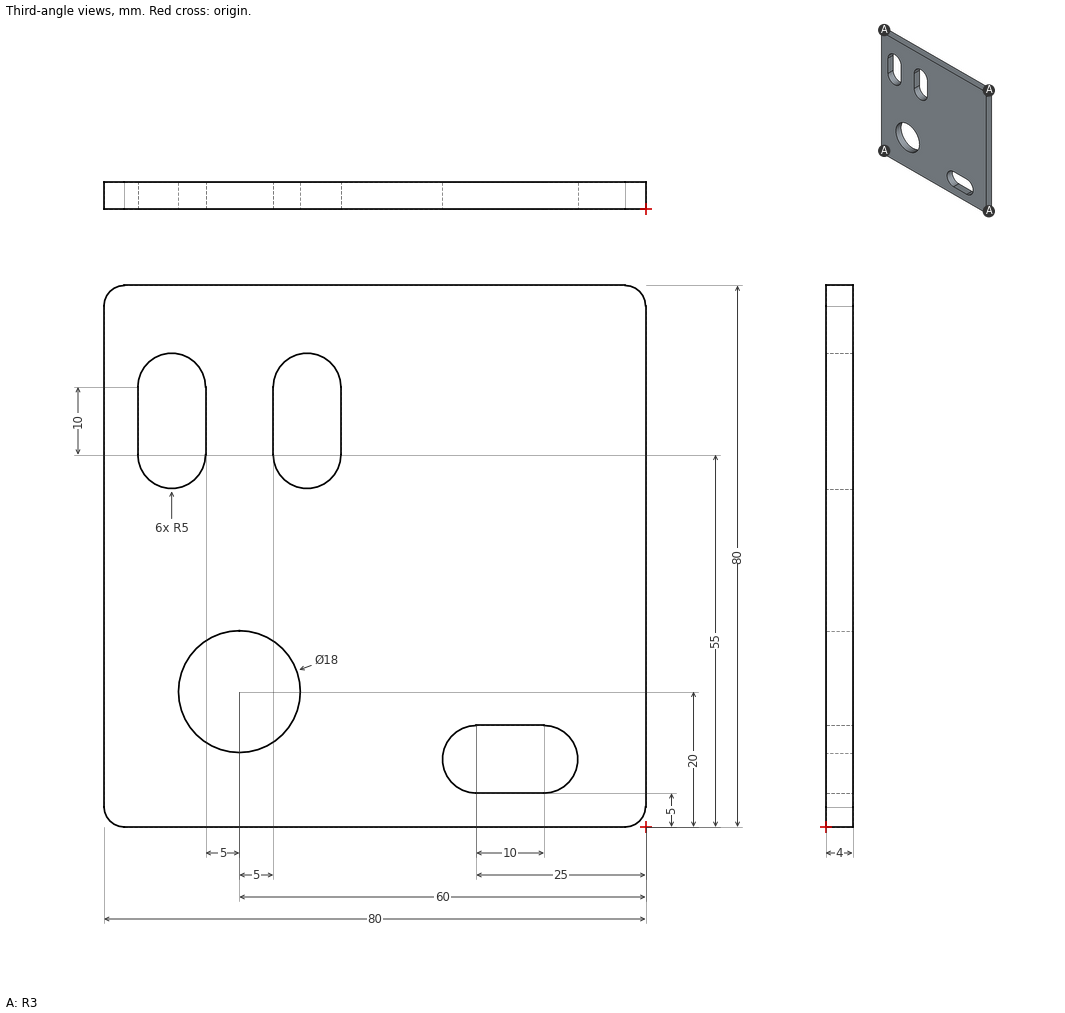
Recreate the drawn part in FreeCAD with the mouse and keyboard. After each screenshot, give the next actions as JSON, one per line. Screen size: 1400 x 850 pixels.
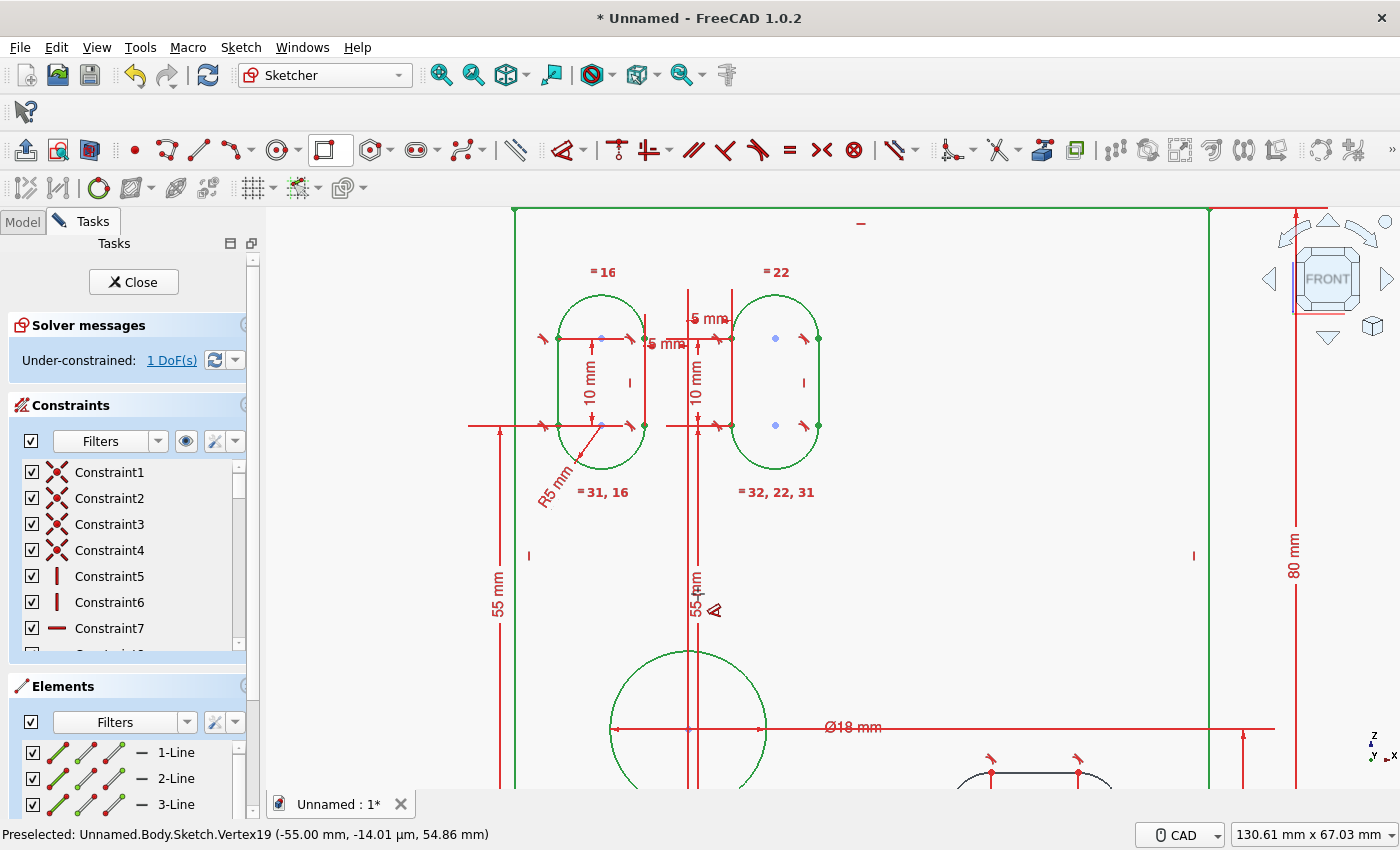
{"action": "scroll", "coordinate": [646, 428], "scroll_direction": "down", "scroll_amount": 3}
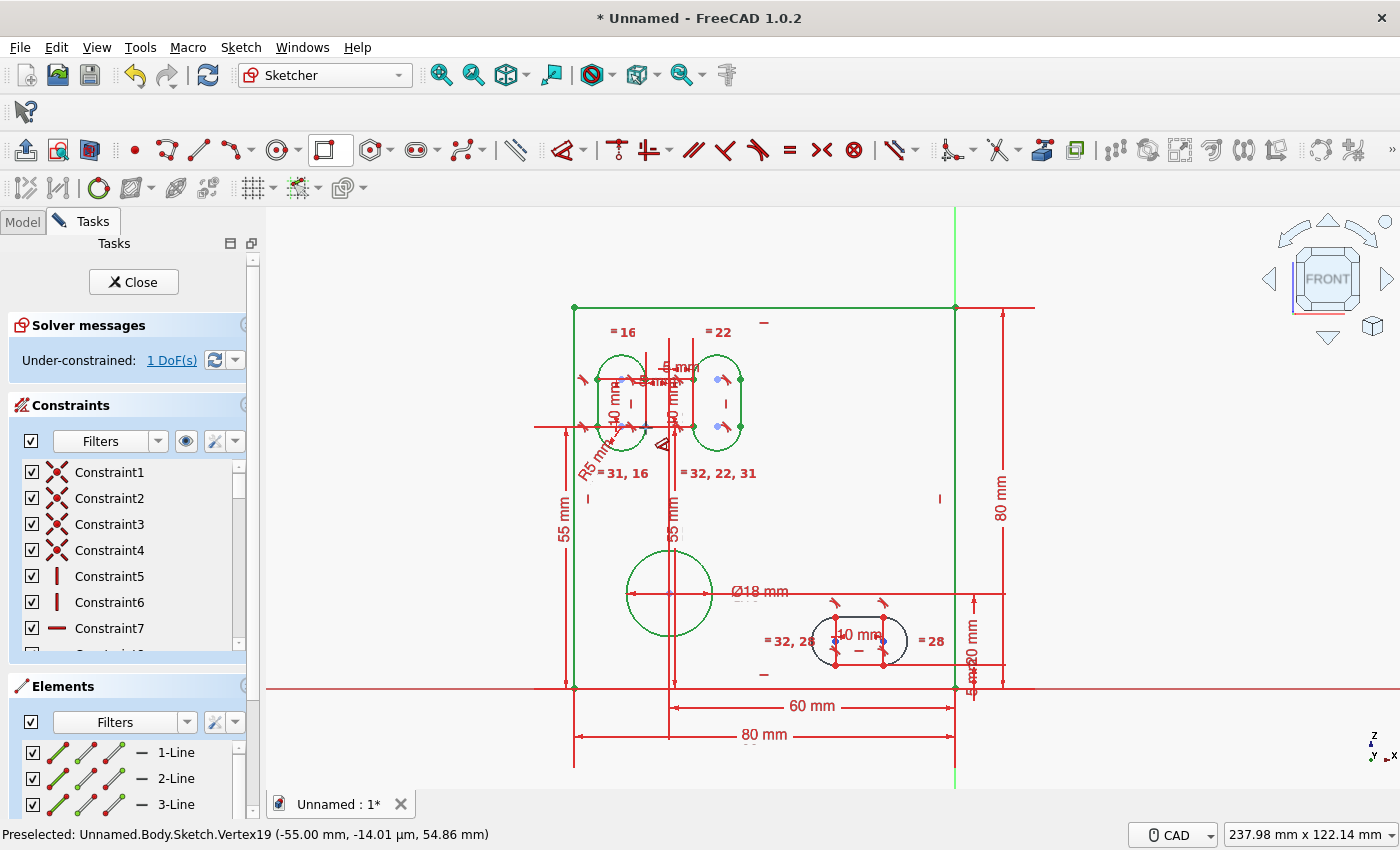
{"action": "left_click", "coordinate": [836, 617]}
{"action": "left_click", "coordinate": [895, 723]}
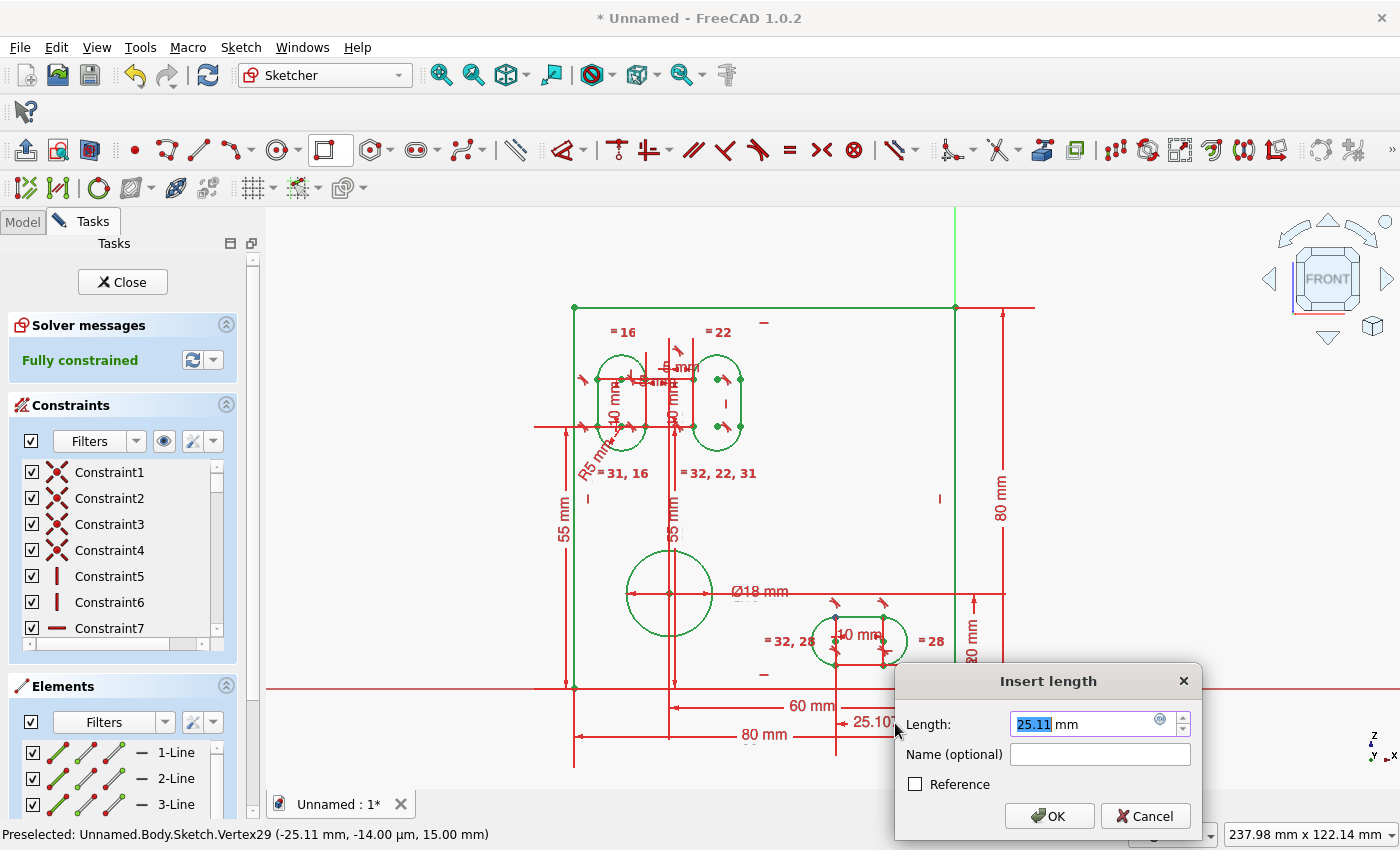
{"action": "type", "text": "25"}
{"action": "key", "text": "Return"}
{"action": "key", "text": "Escape"}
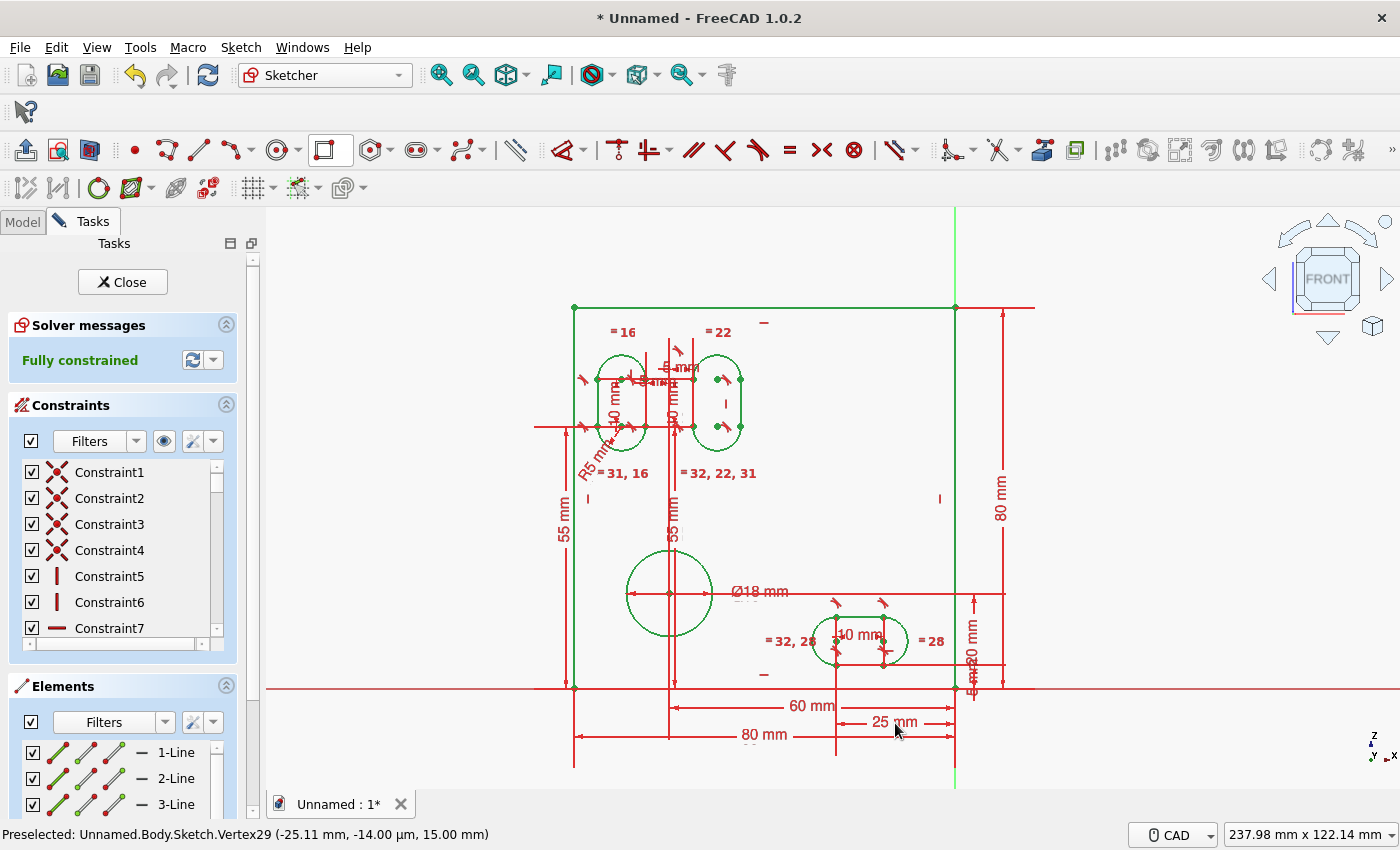
{"action": "left_click", "coordinate": [123, 282]}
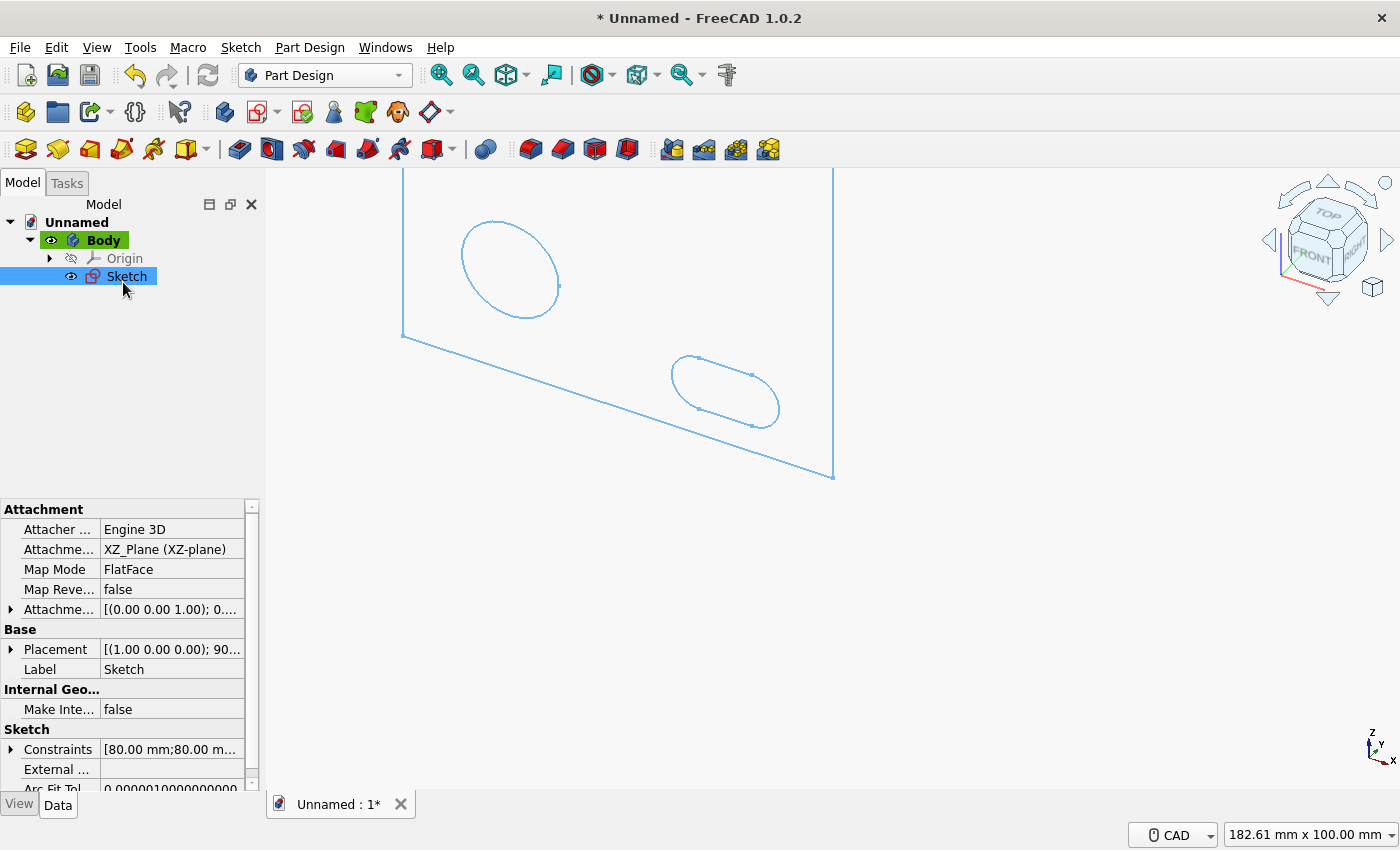
{"action": "left_click", "coordinate": [26, 150]}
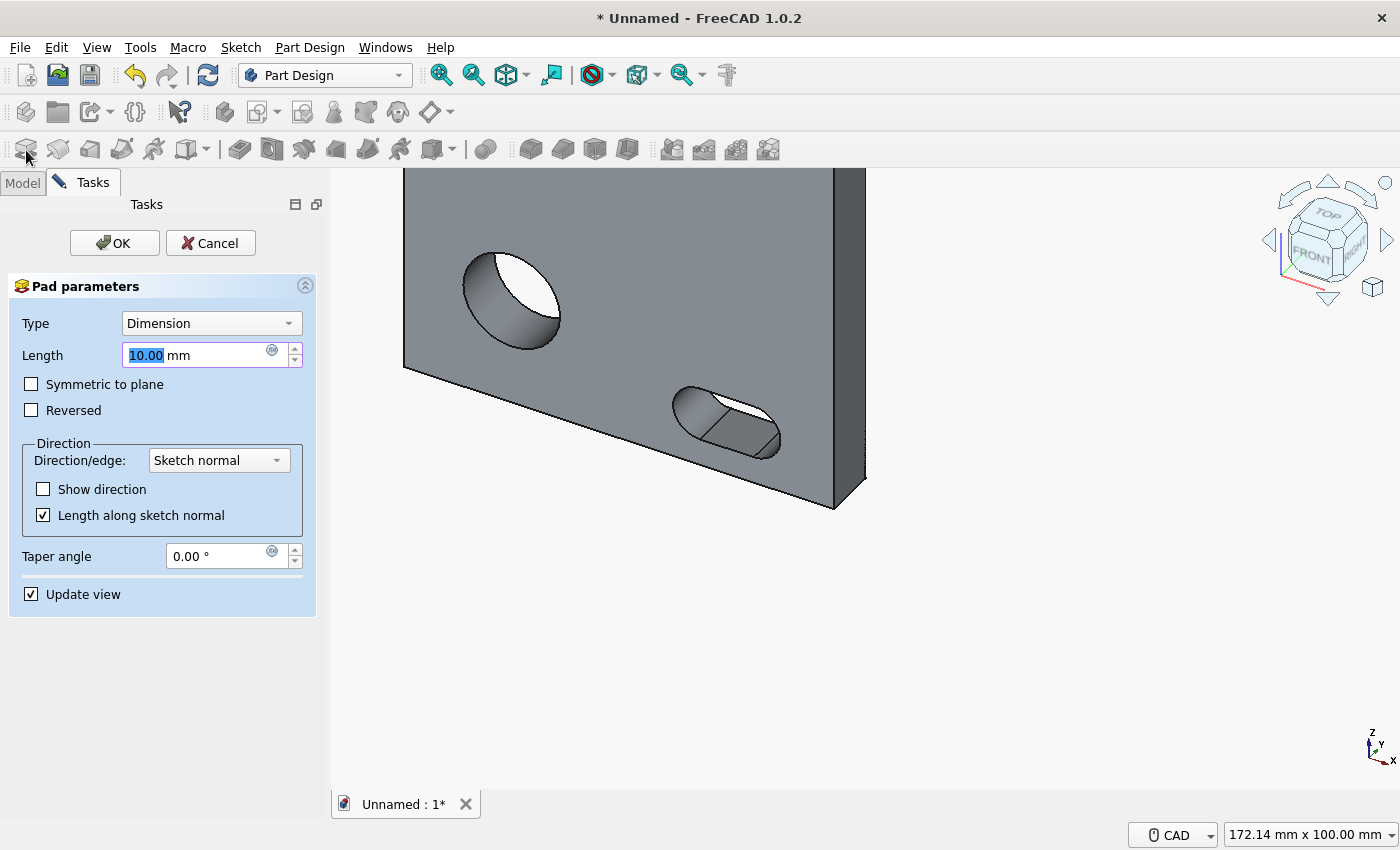
{"action": "type", "text": "4"}
{"action": "key", "text": "Tab"}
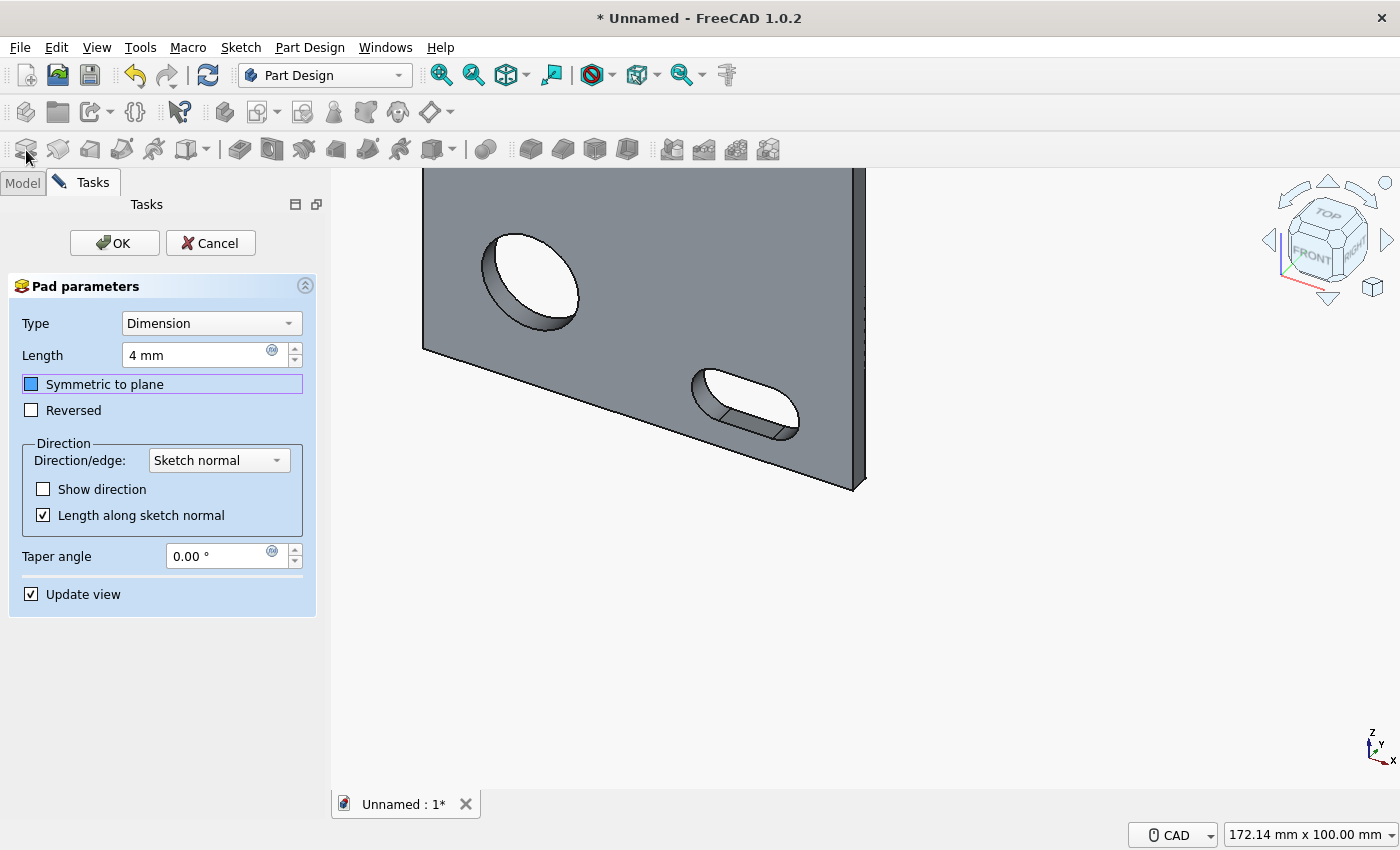
{"action": "left_click", "coordinate": [30, 410]}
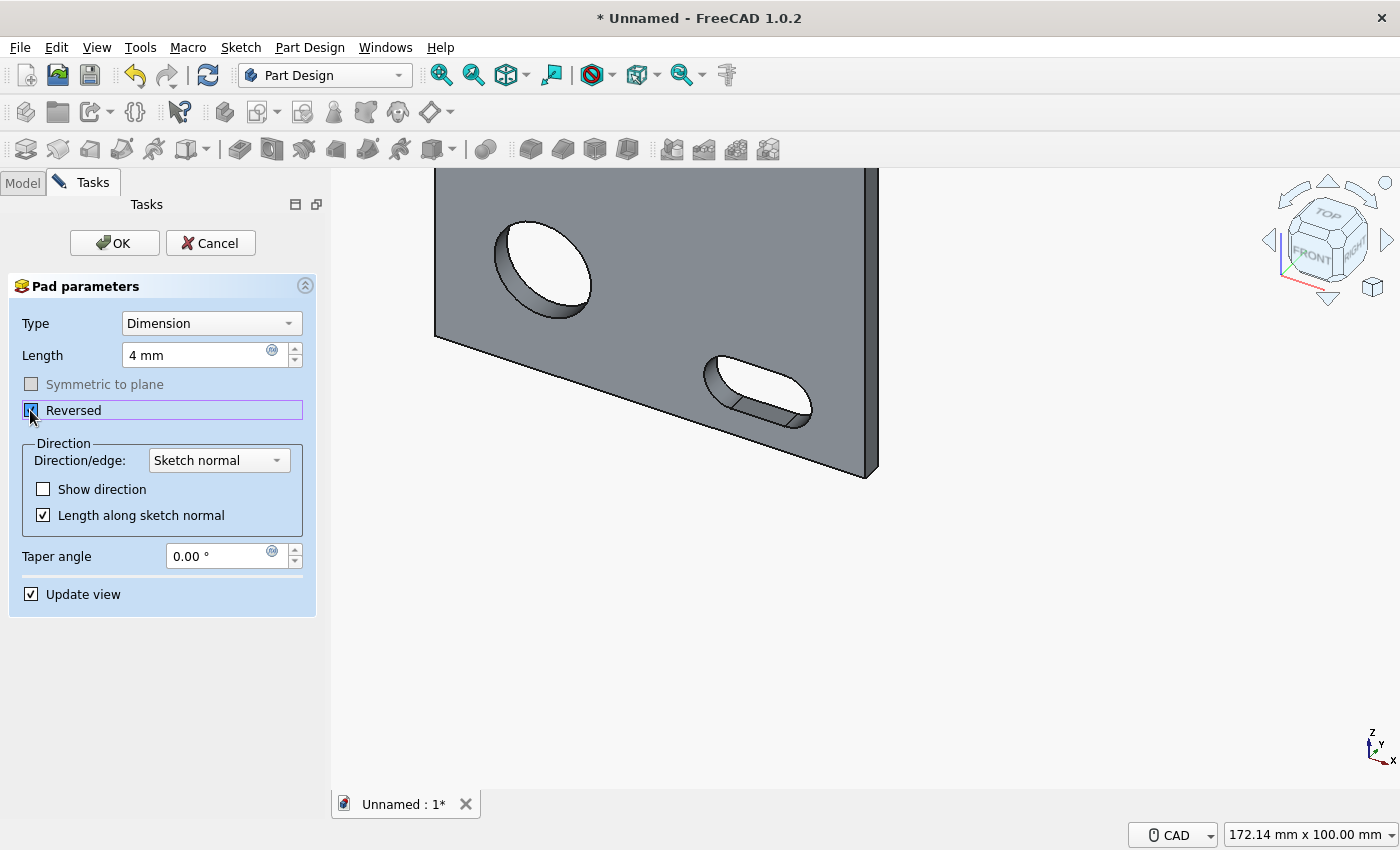
{"action": "left_click", "coordinate": [115, 243]}